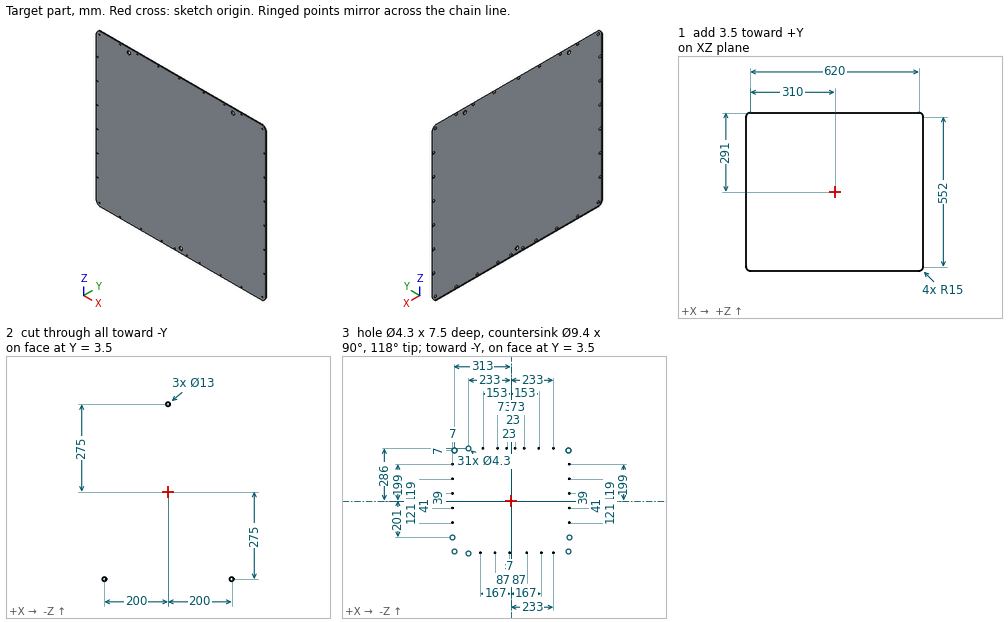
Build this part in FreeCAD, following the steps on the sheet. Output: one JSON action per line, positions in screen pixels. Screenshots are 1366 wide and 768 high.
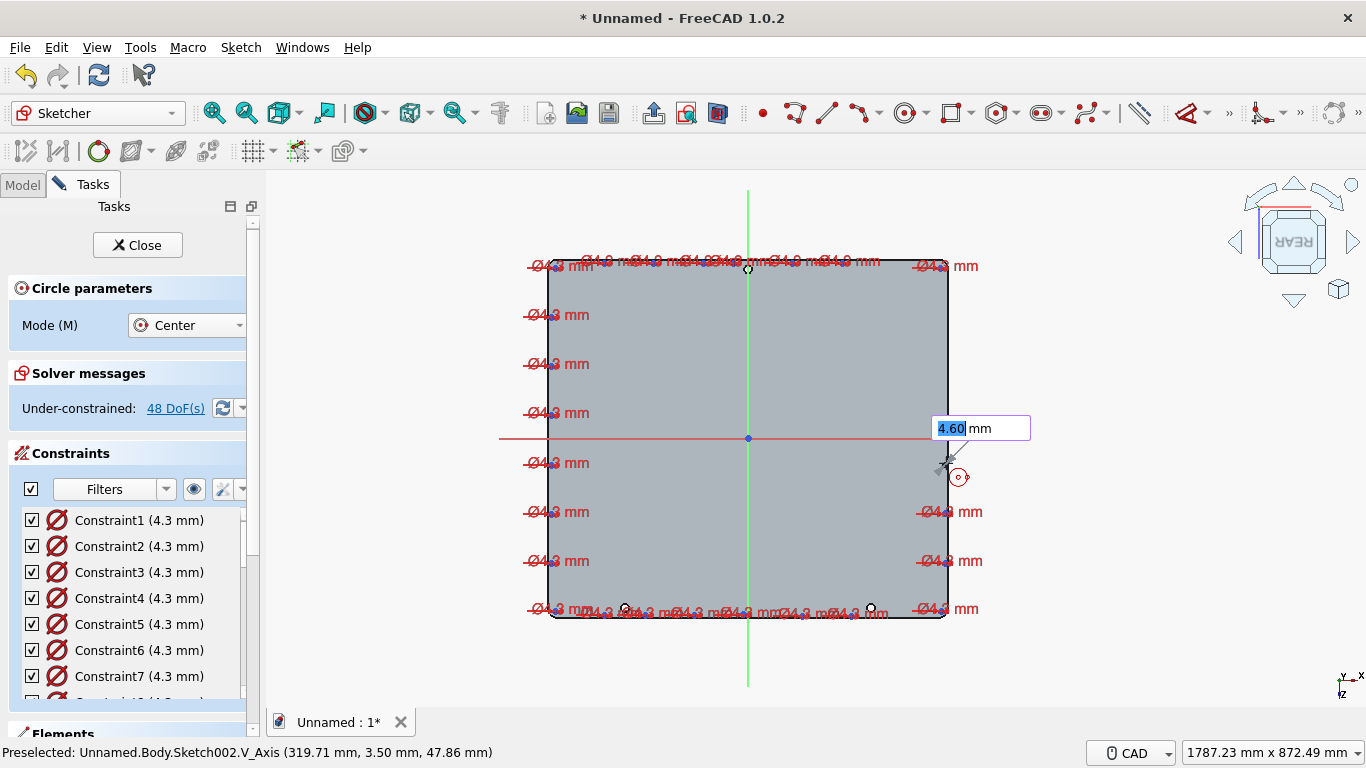
{"action": "type", "text": "4.3"}
{"action": "key", "text": "Return"}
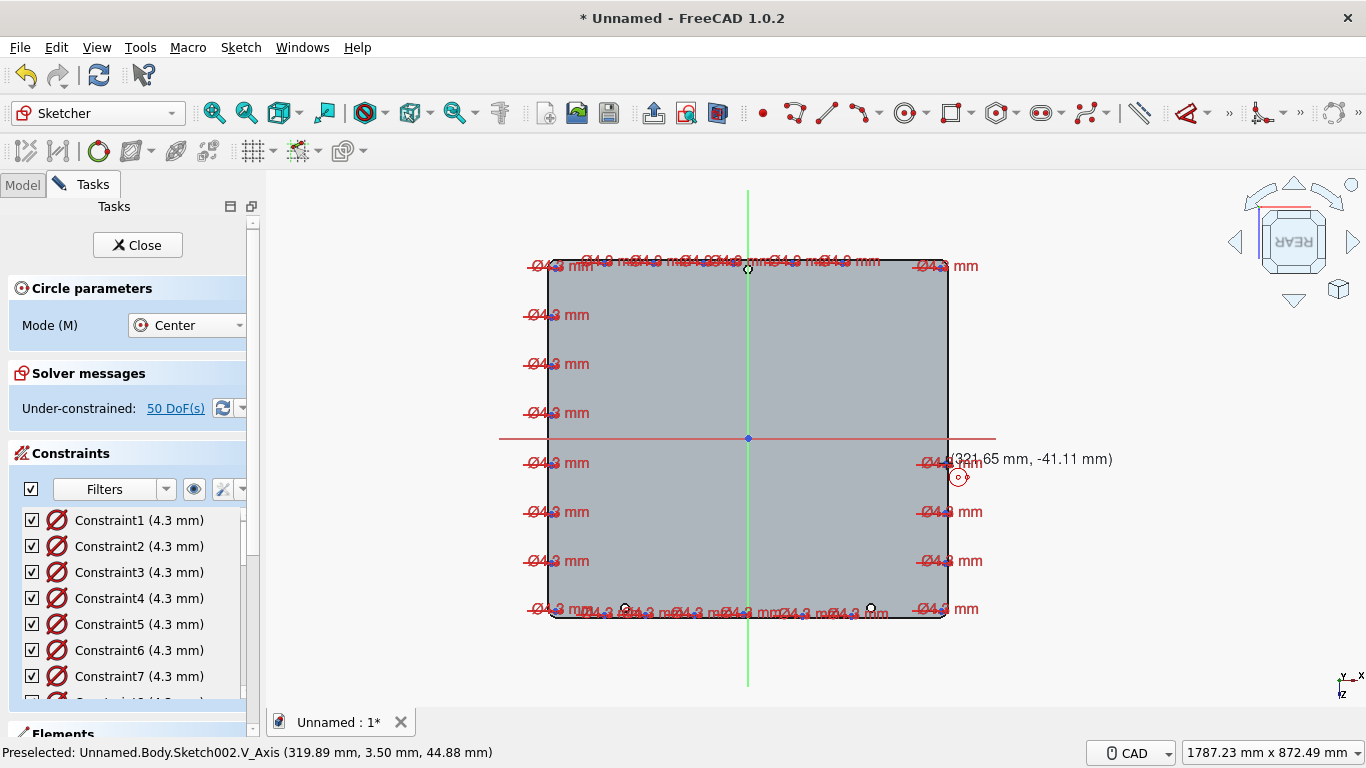
{"action": "scroll", "coordinate": [945, 415], "scroll_direction": "up", "scroll_amount": 15}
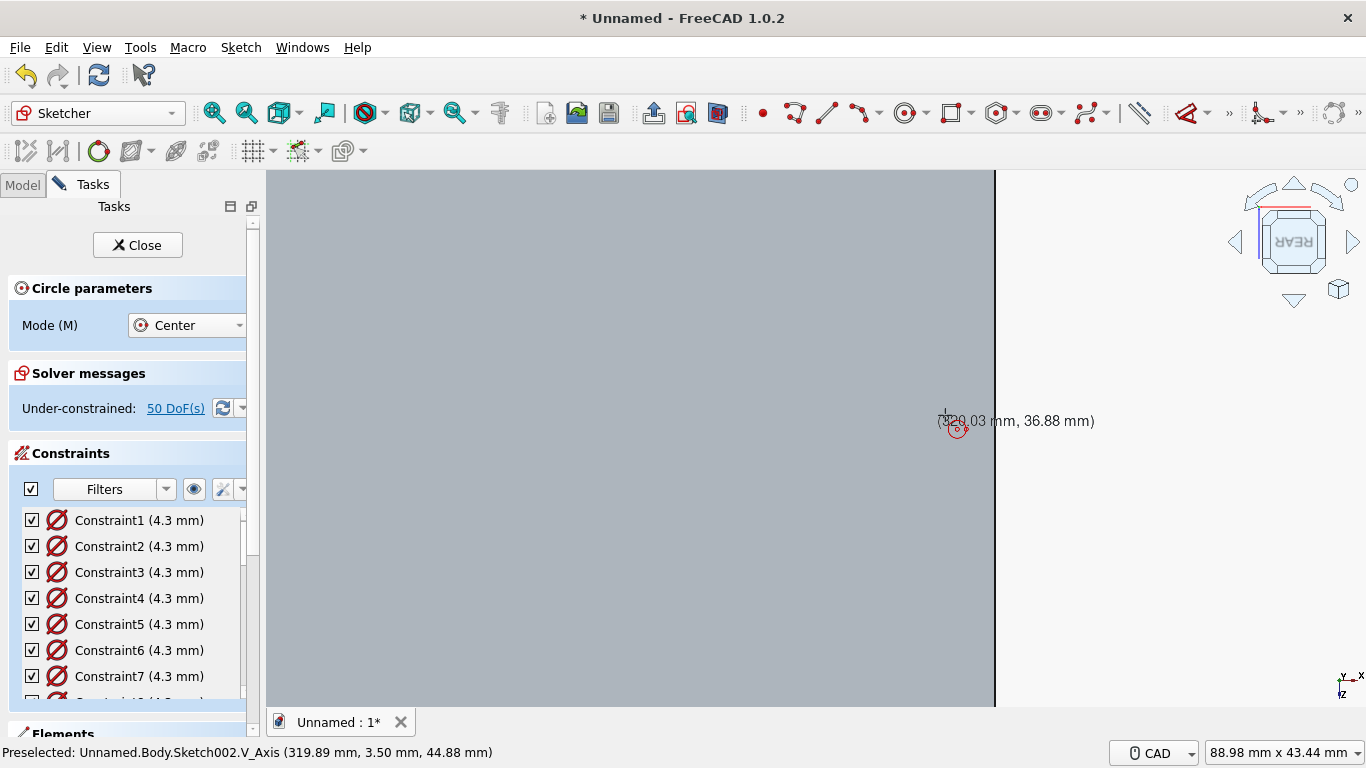
{"action": "scroll", "coordinate": [945, 415], "scroll_direction": "down", "scroll_amount": 15}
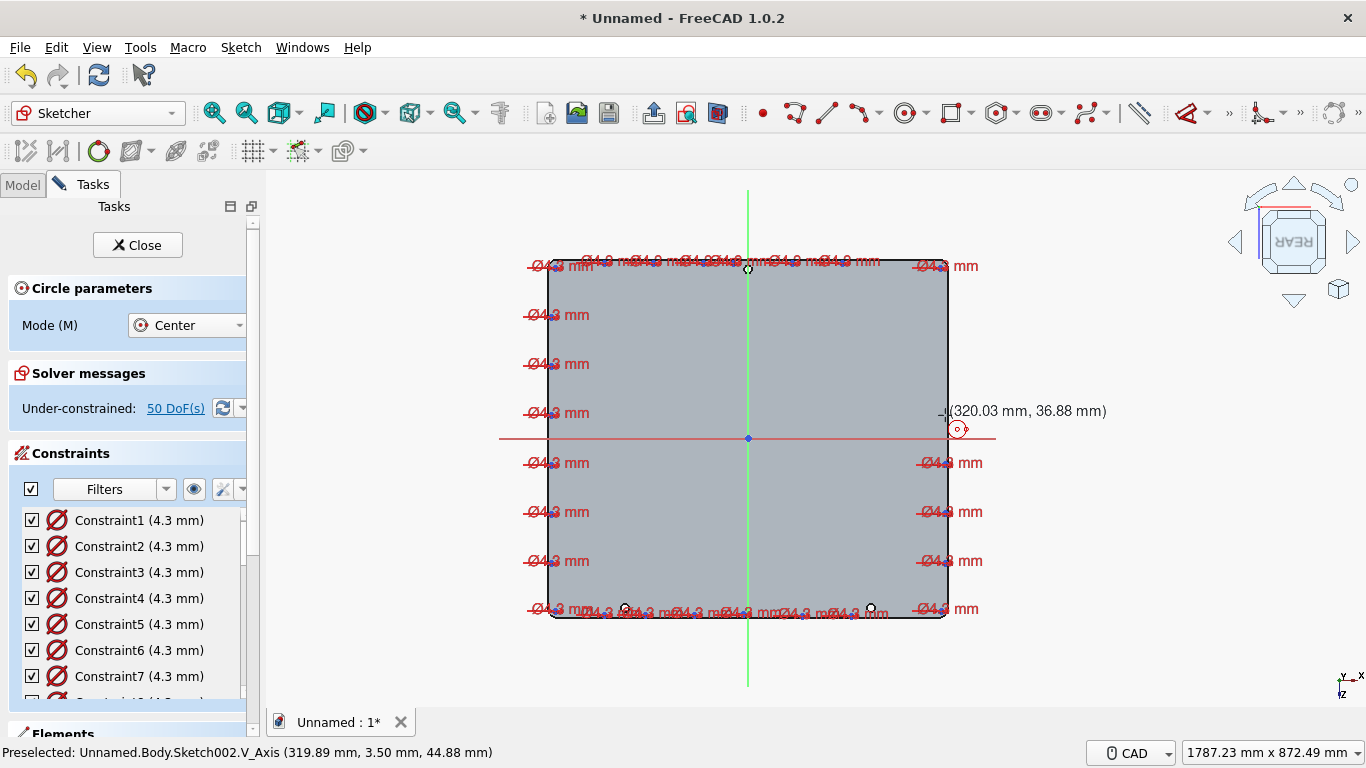
{"action": "left_click", "coordinate": [945, 415]}
{"action": "mouse_move", "coordinate": [946, 414]}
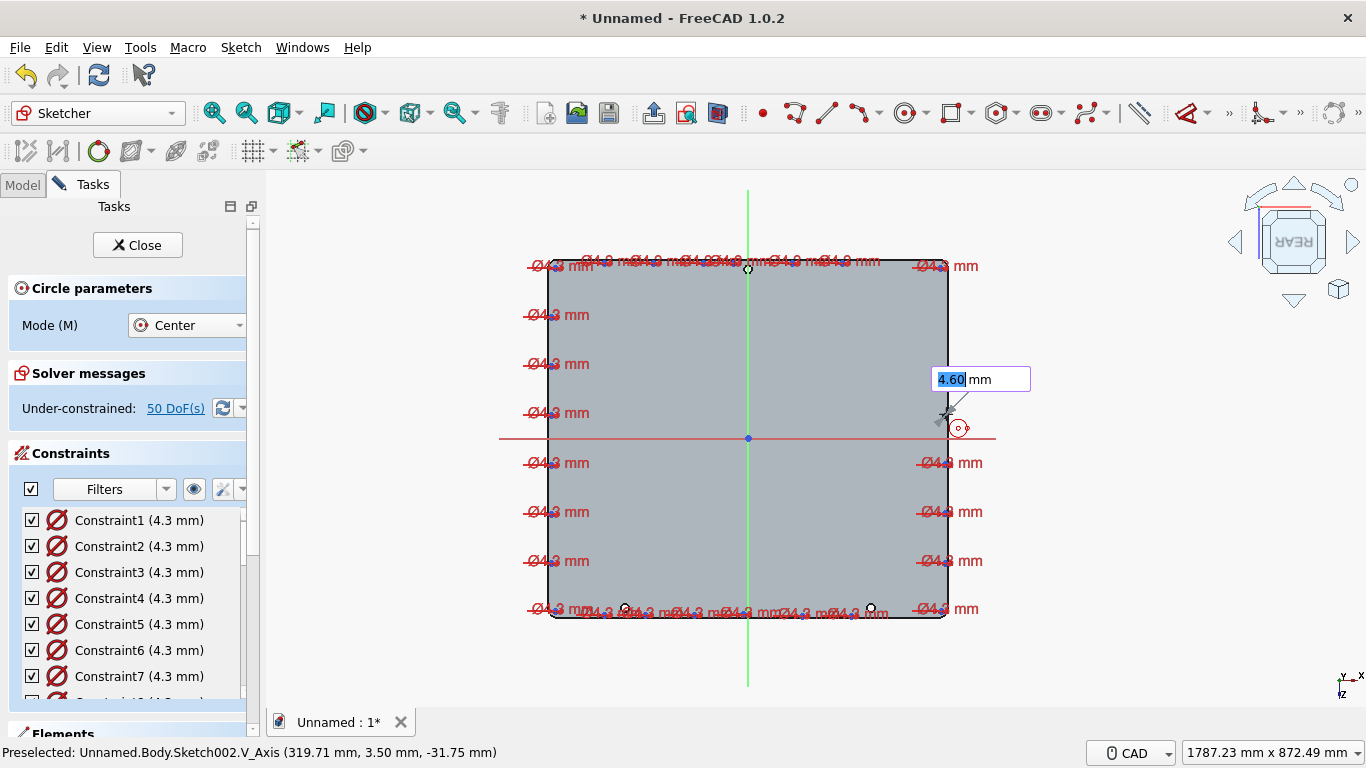
{"action": "type", "text": "4.3"}
{"action": "key", "text": "Return"}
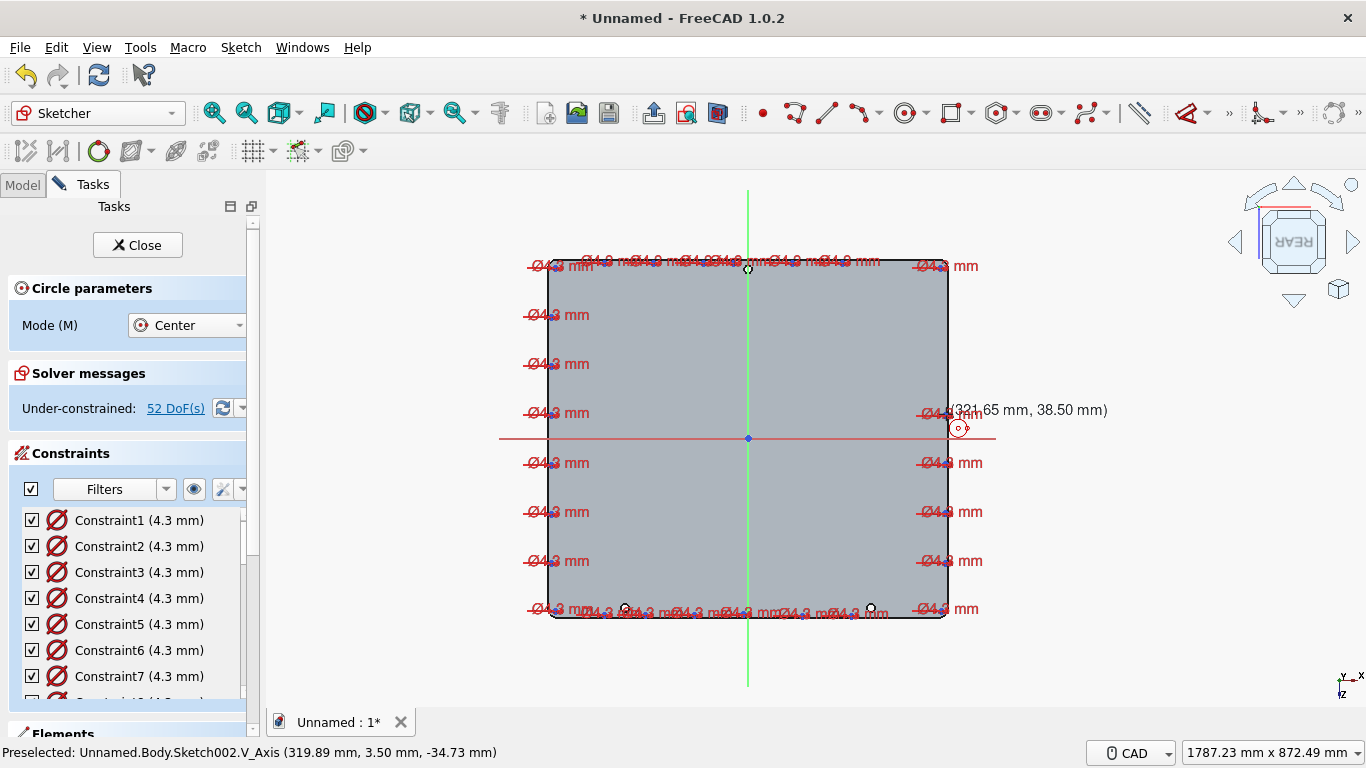
{"action": "scroll", "coordinate": [945, 365], "scroll_direction": "up", "scroll_amount": 15}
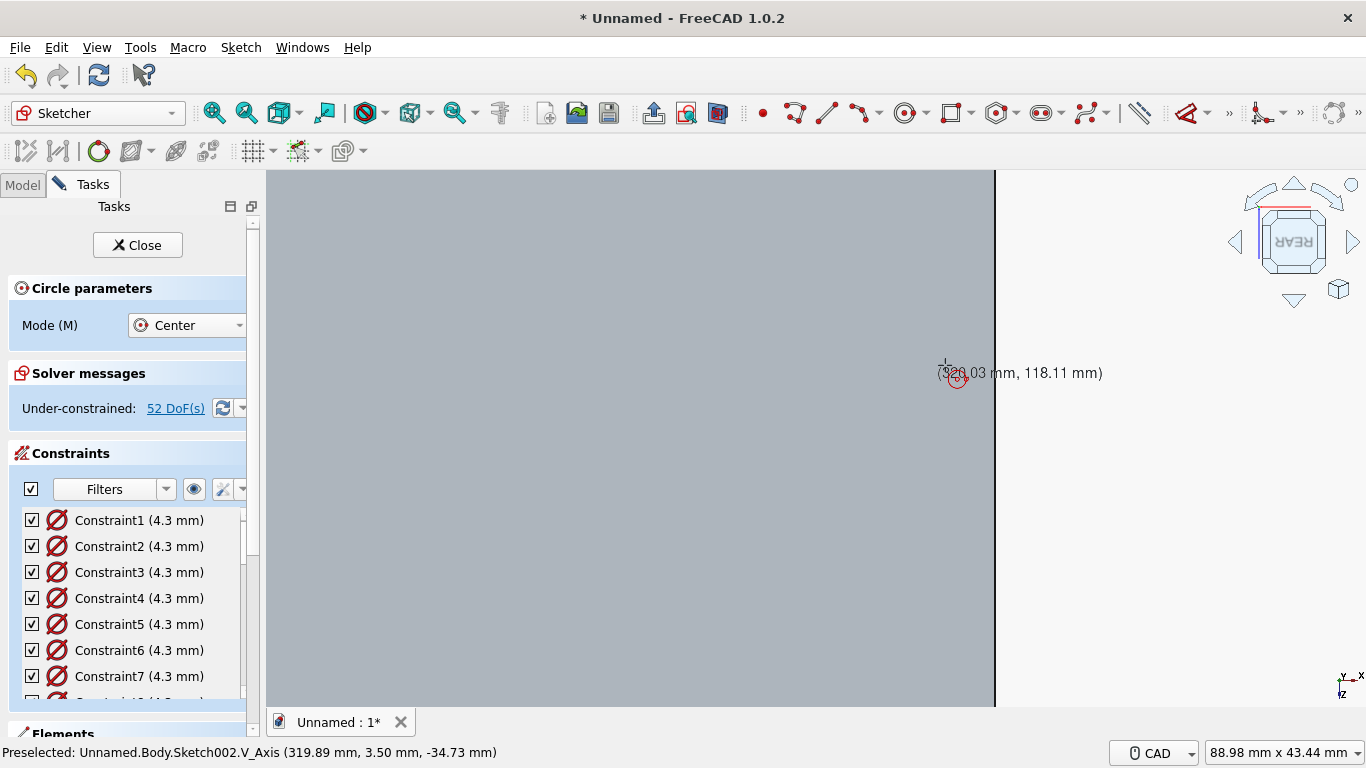
{"action": "scroll", "coordinate": [945, 365], "scroll_direction": "down", "scroll_amount": 15}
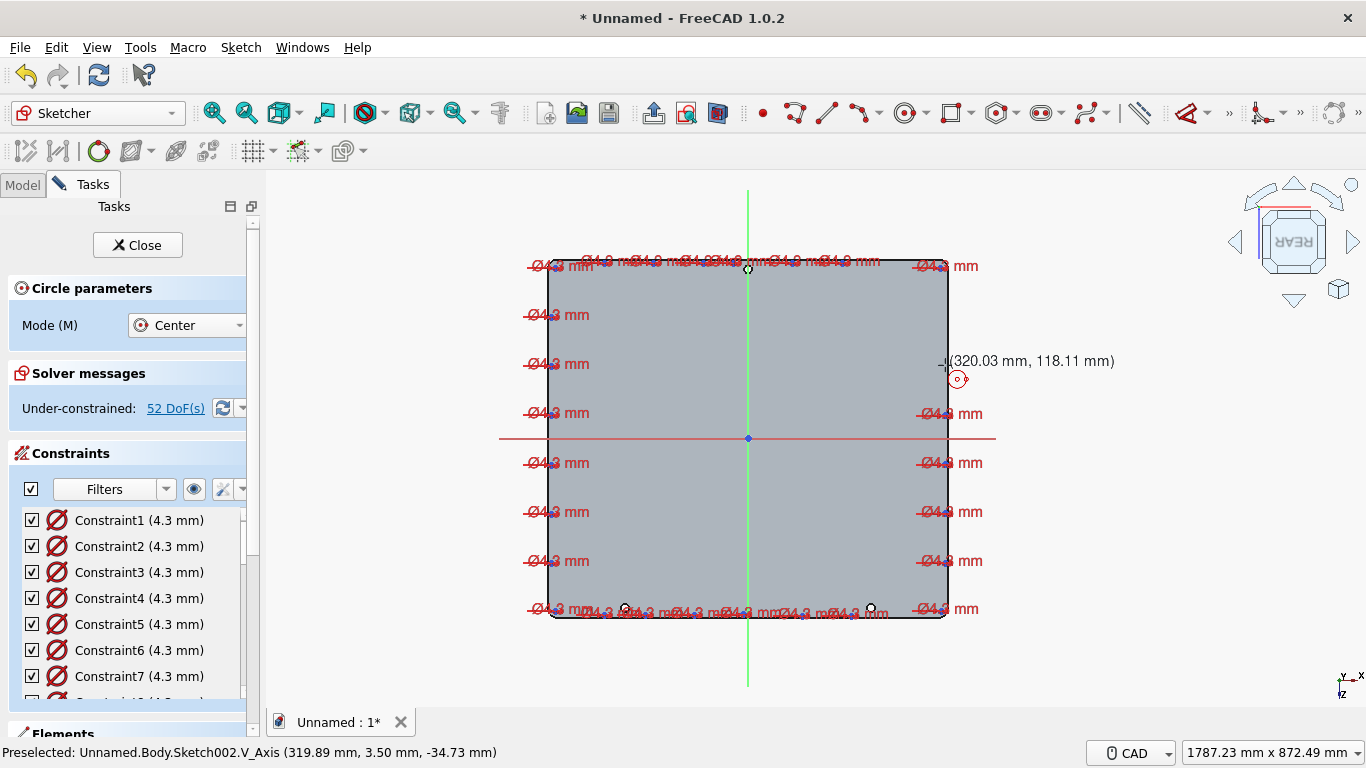
{"action": "left_click", "coordinate": [945, 365]}
{"action": "mouse_move", "coordinate": [946, 365]}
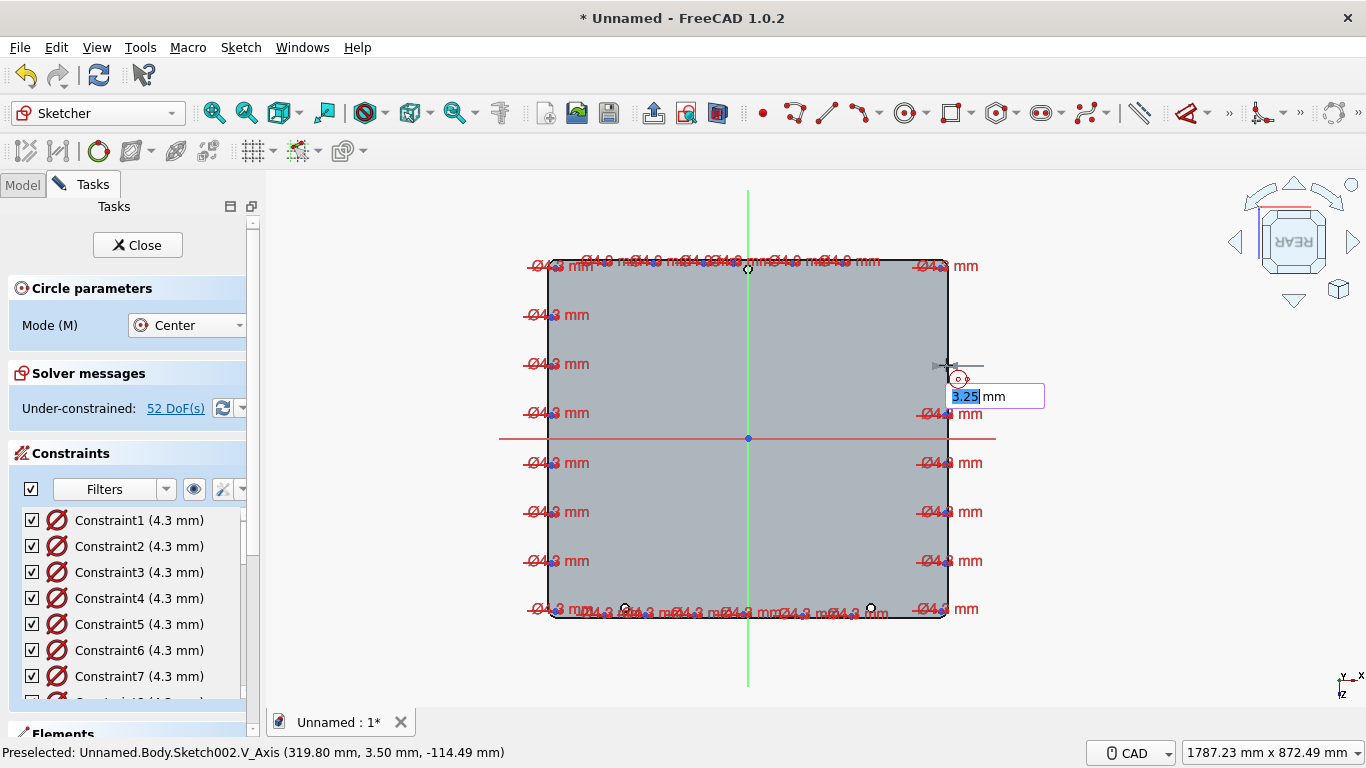
{"action": "type", "text": "4.3"}
{"action": "key", "text": "Return"}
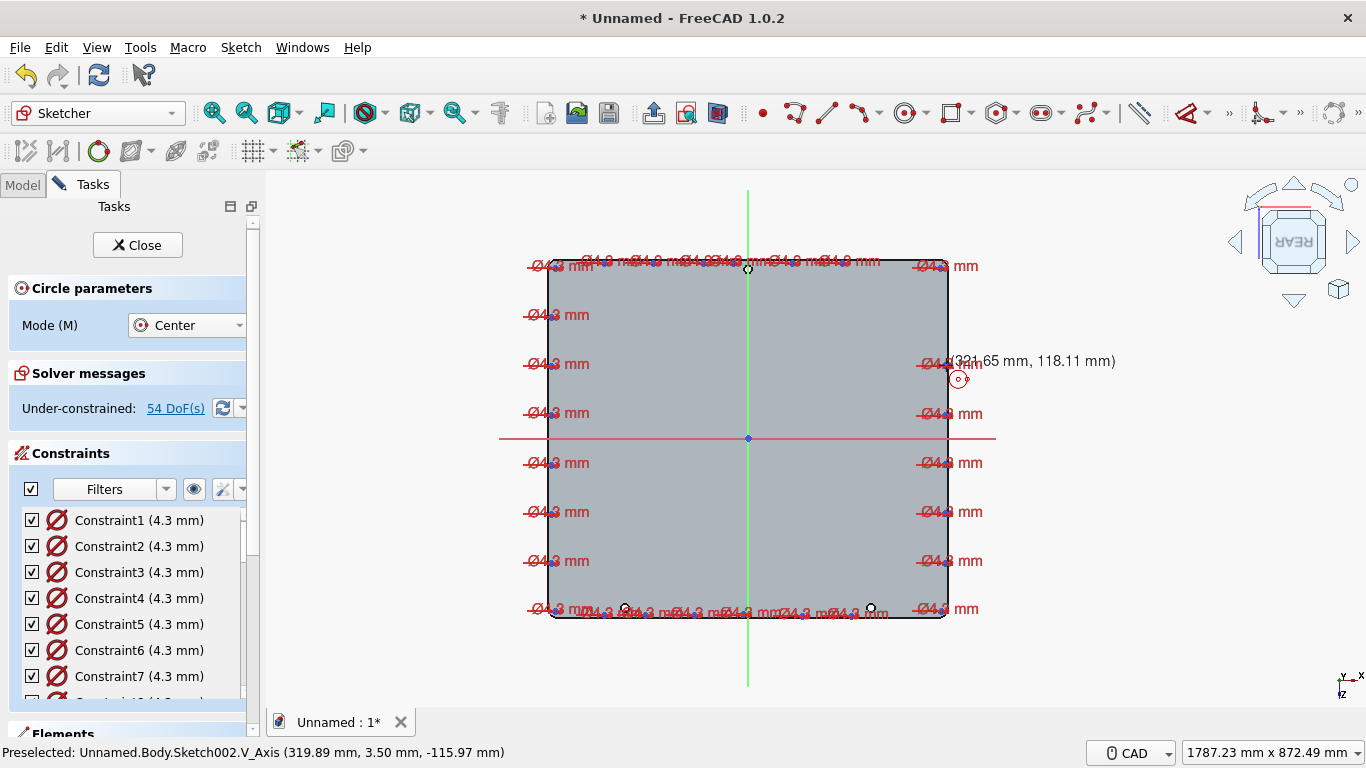
{"action": "scroll", "coordinate": [945, 316], "scroll_direction": "up", "scroll_amount": 15}